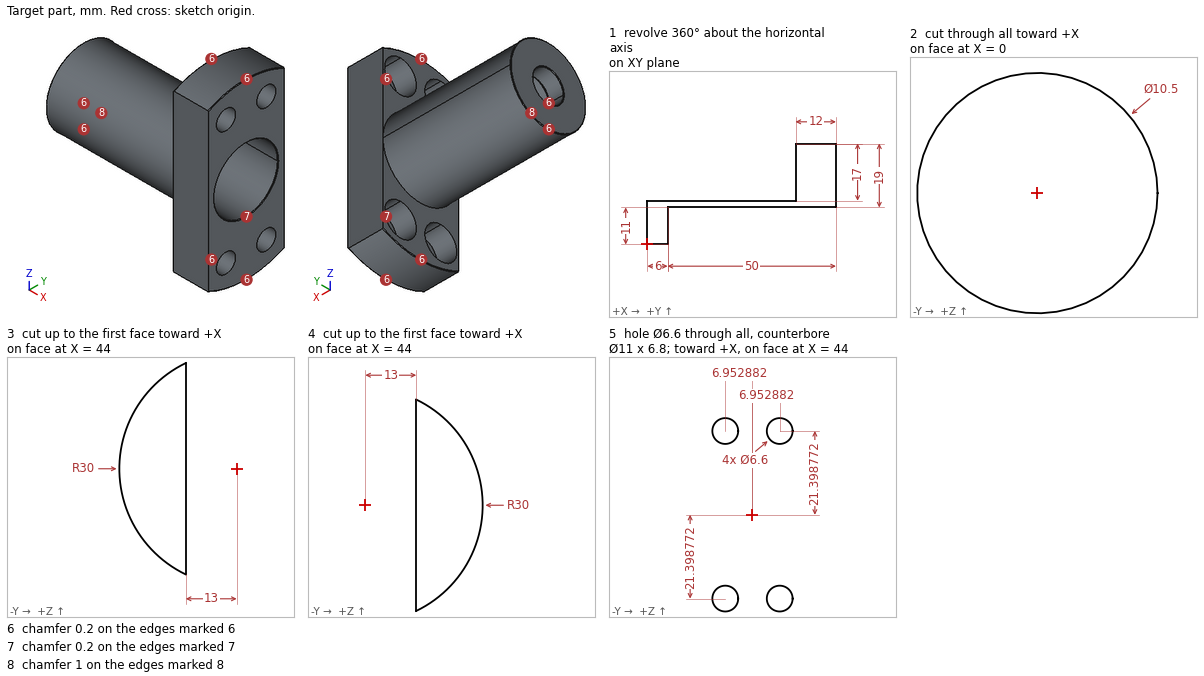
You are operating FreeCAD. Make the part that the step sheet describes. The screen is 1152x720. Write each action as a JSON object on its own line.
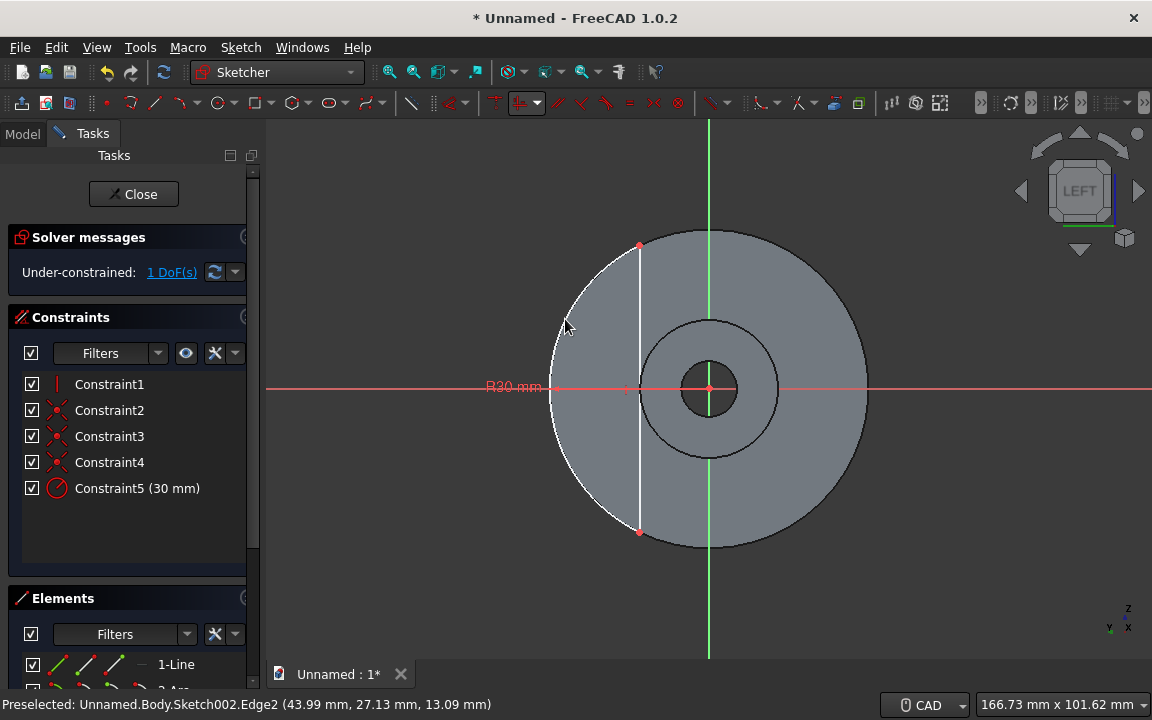
{"action": "left_click", "coordinate": [640, 533]}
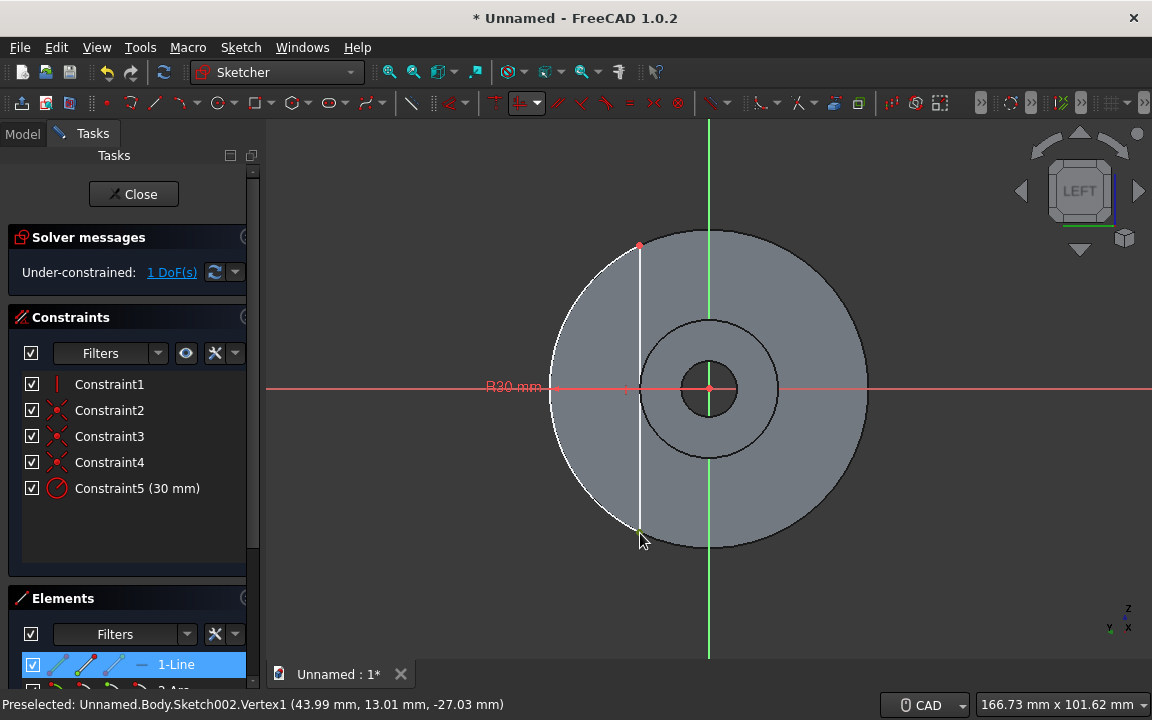
{"action": "key", "text": "l"}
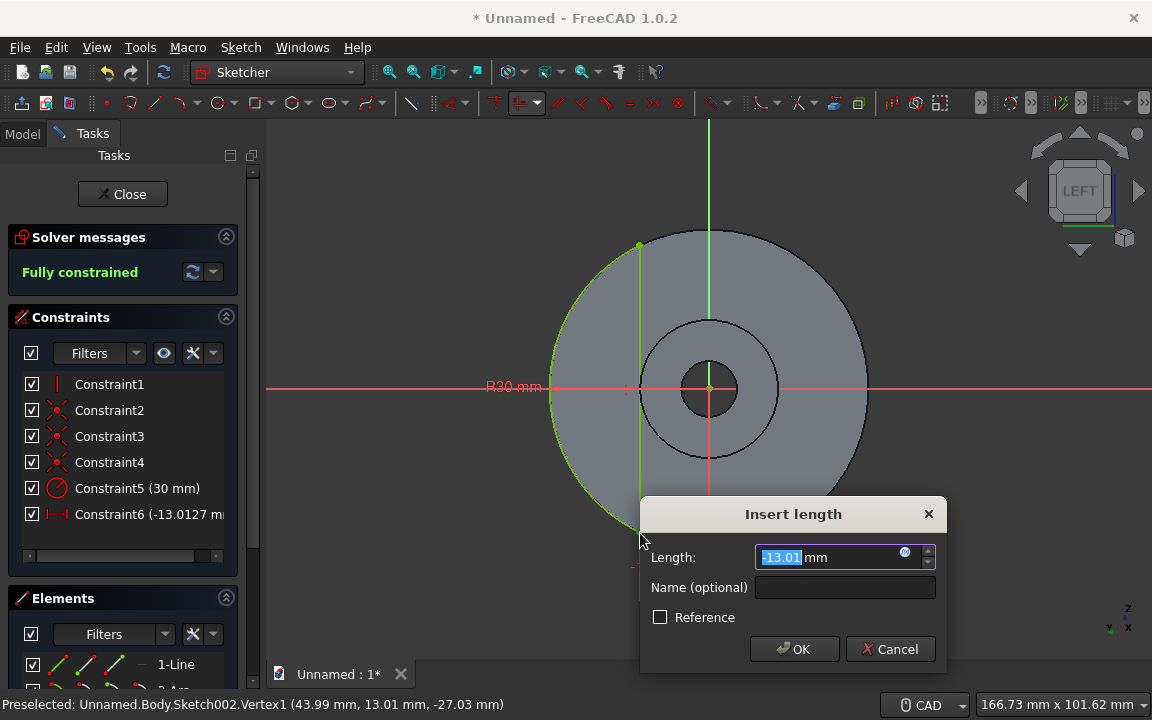
{"action": "type", "text": "-13"}
{"action": "key", "text": "Return"}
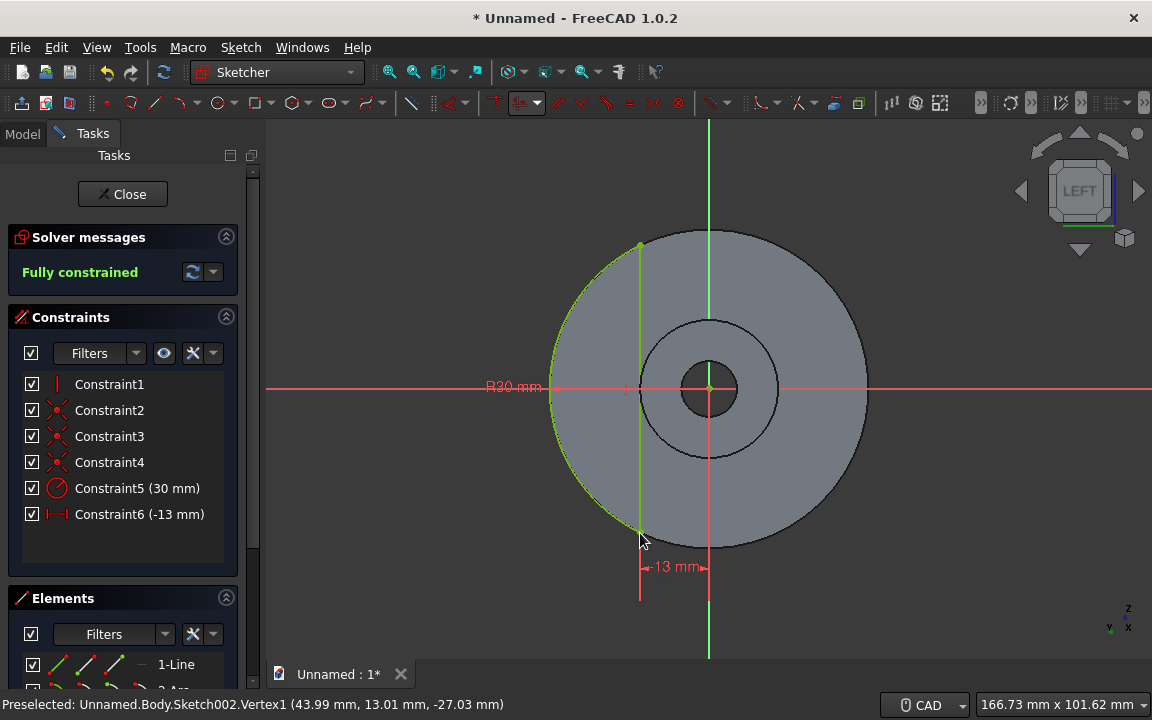
{"action": "left_click", "coordinate": [123, 194]}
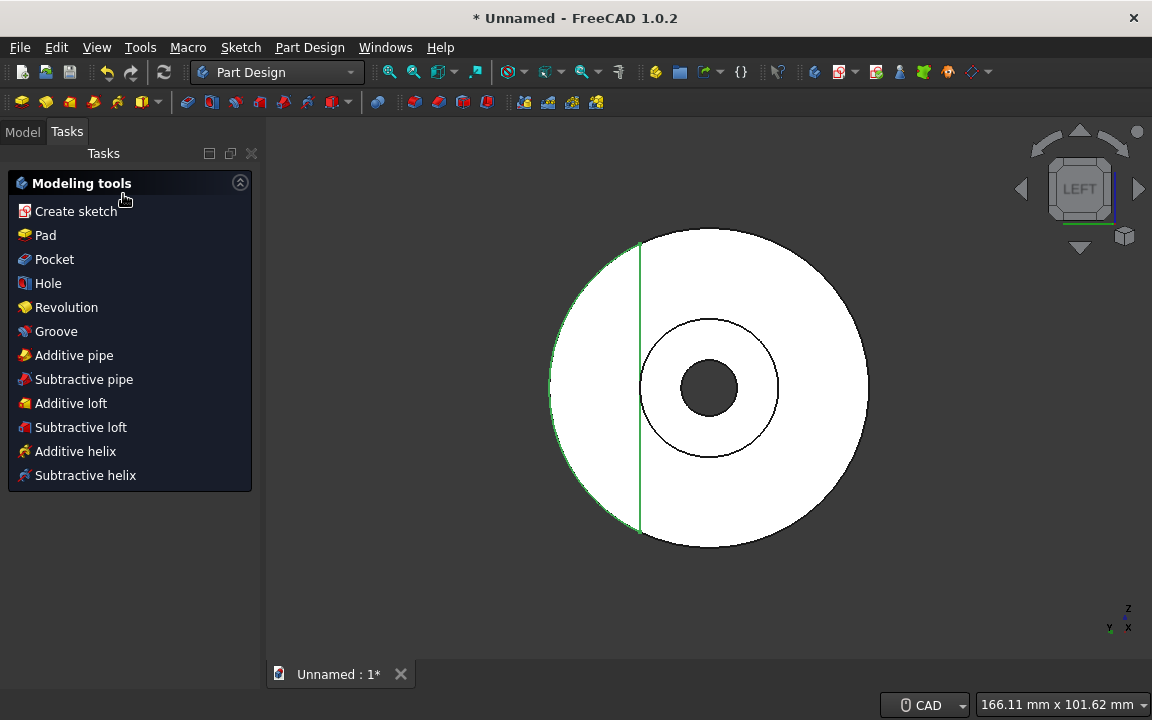
{"action": "left_click", "coordinate": [188, 102]}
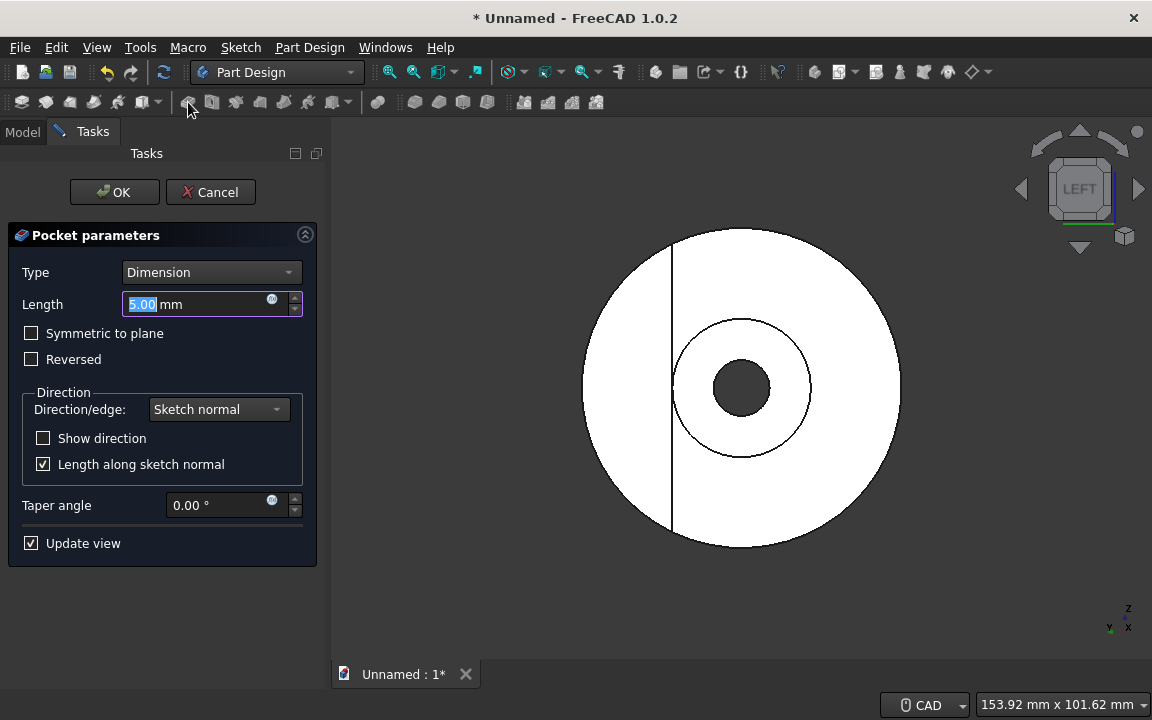
{"action": "left_click", "coordinate": [212, 272]}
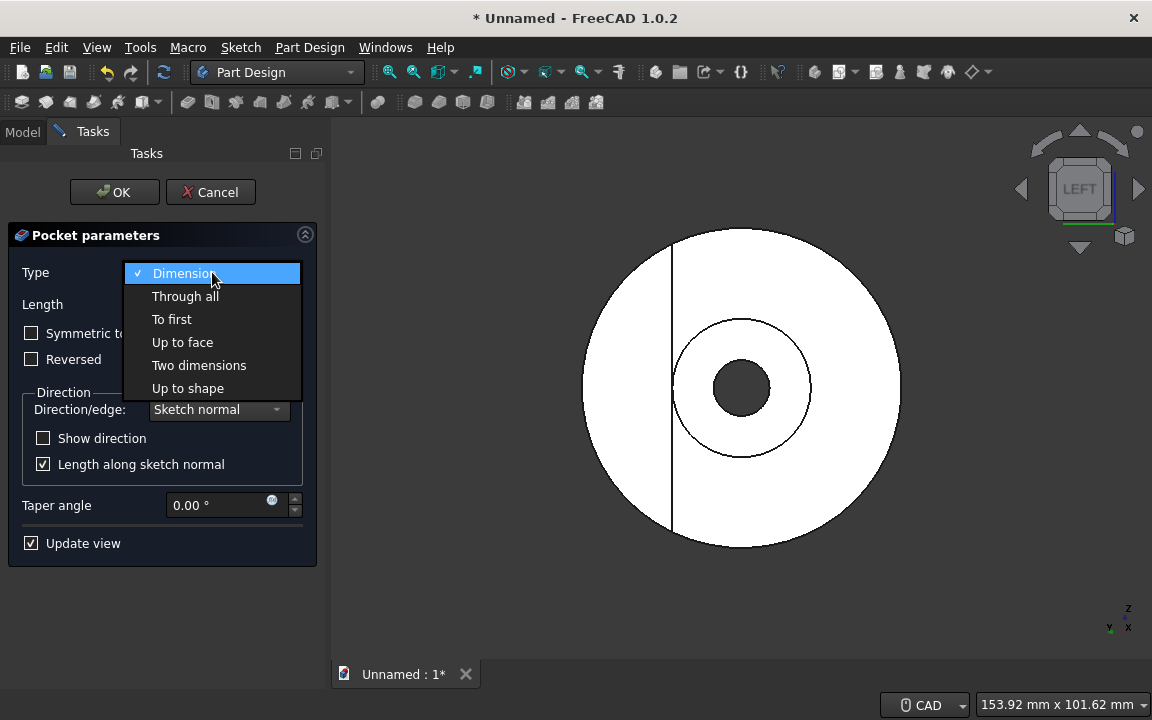
{"action": "left_click", "coordinate": [212, 320]}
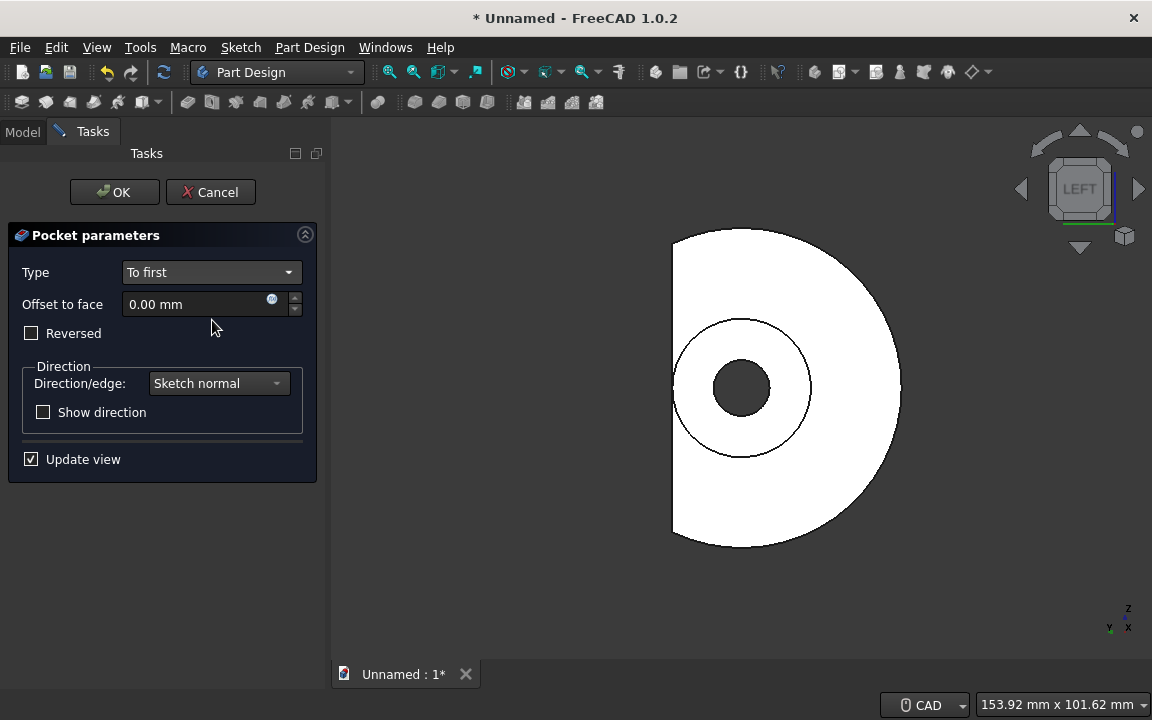
{"action": "left_click", "coordinate": [115, 192]}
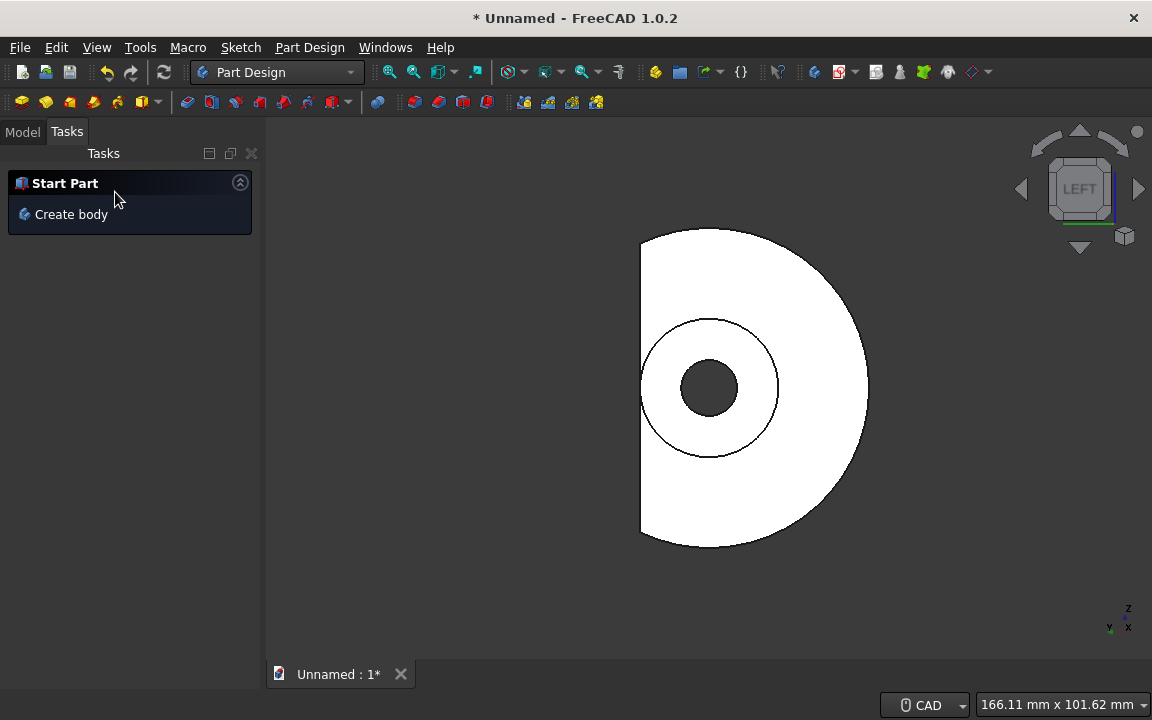
{"action": "left_click", "coordinate": [820, 387]}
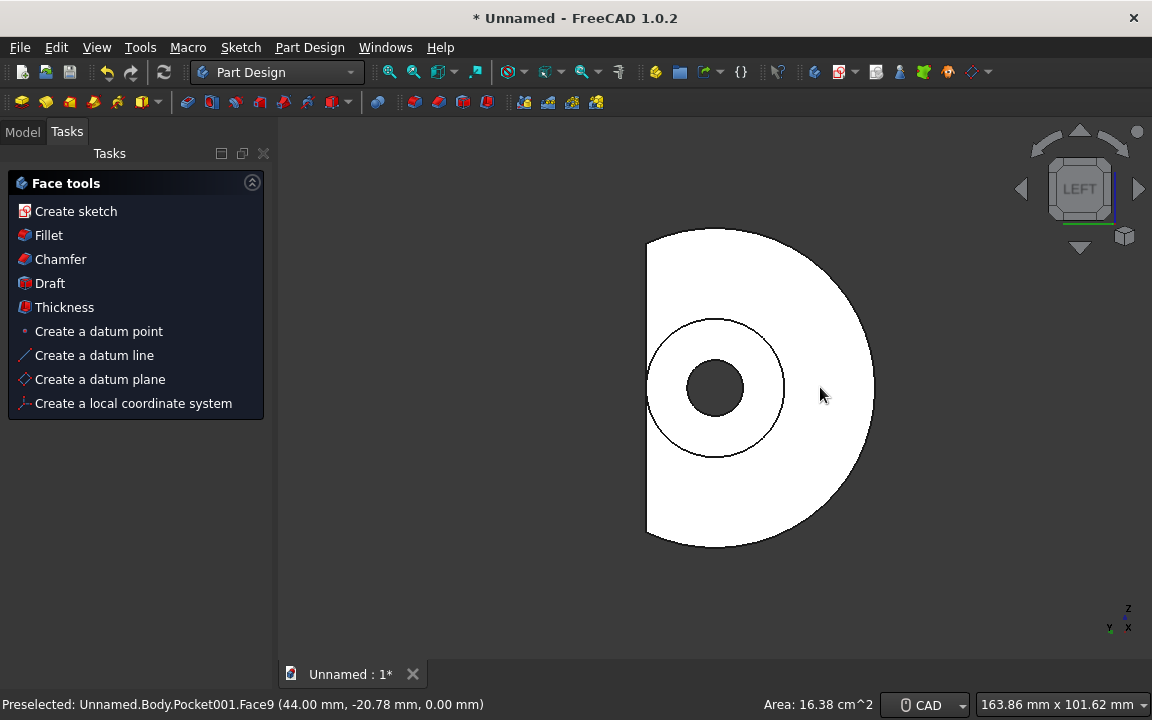
{"action": "left_click", "coordinate": [840, 72]}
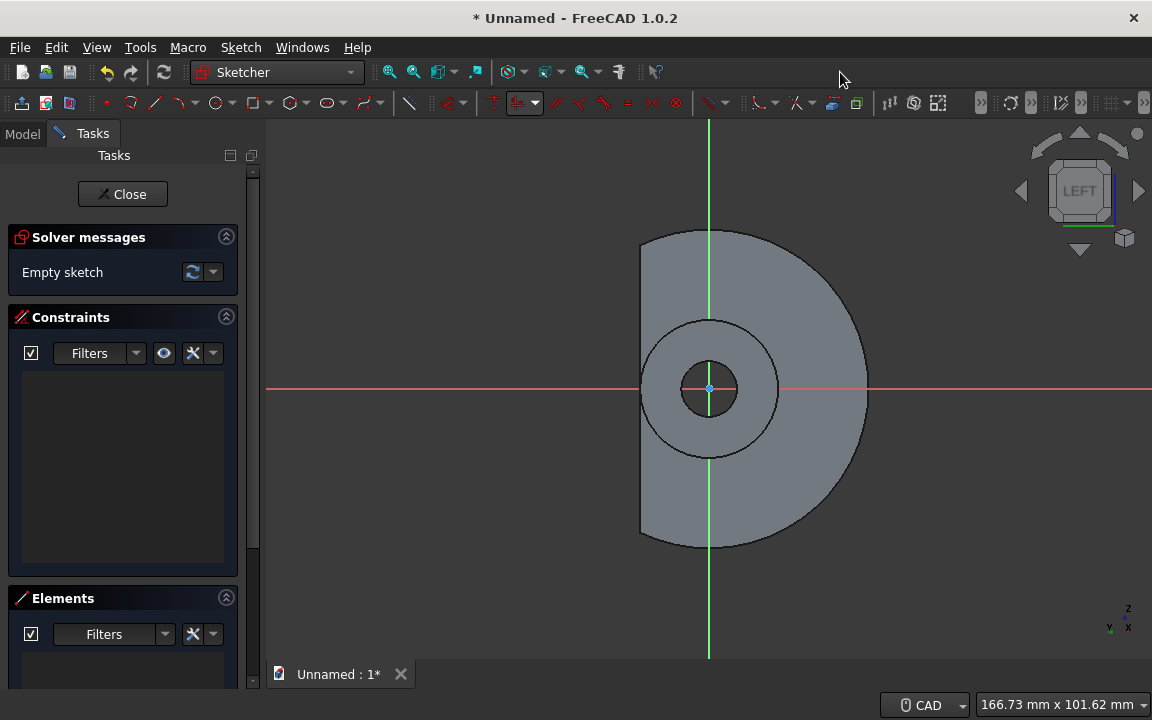
{"action": "key", "text": "g l"}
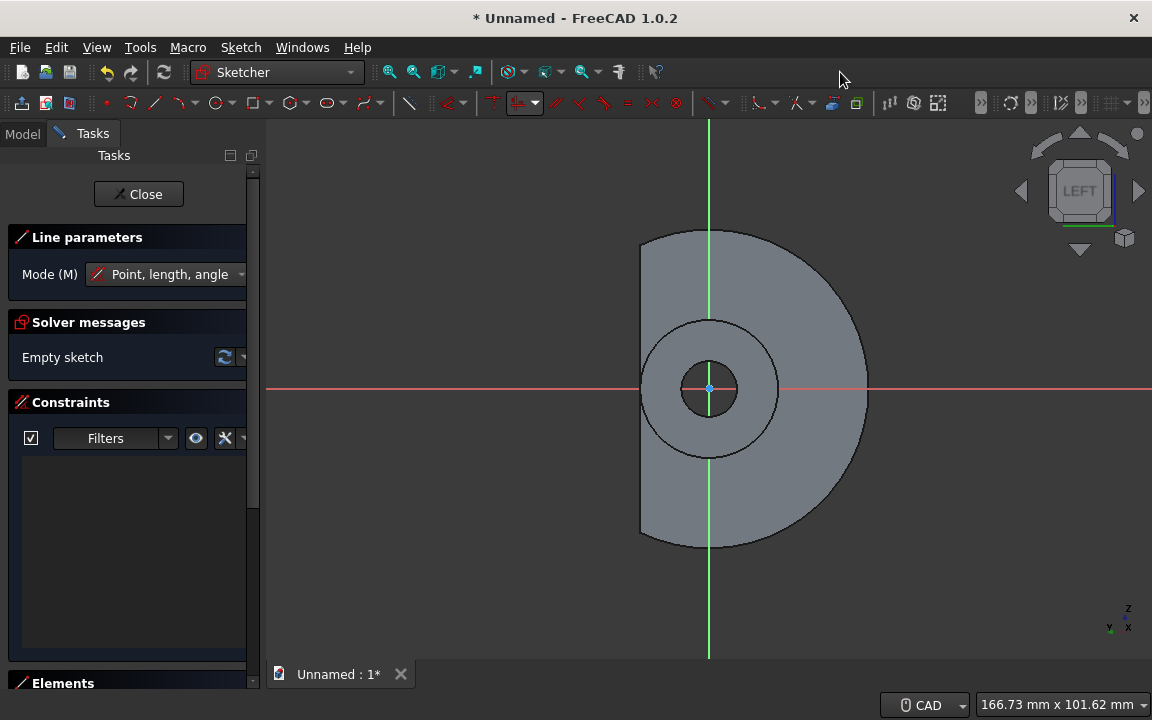
{"action": "left_click", "coordinate": [778, 245]}
{"action": "left_click", "coordinate": [778, 533]}